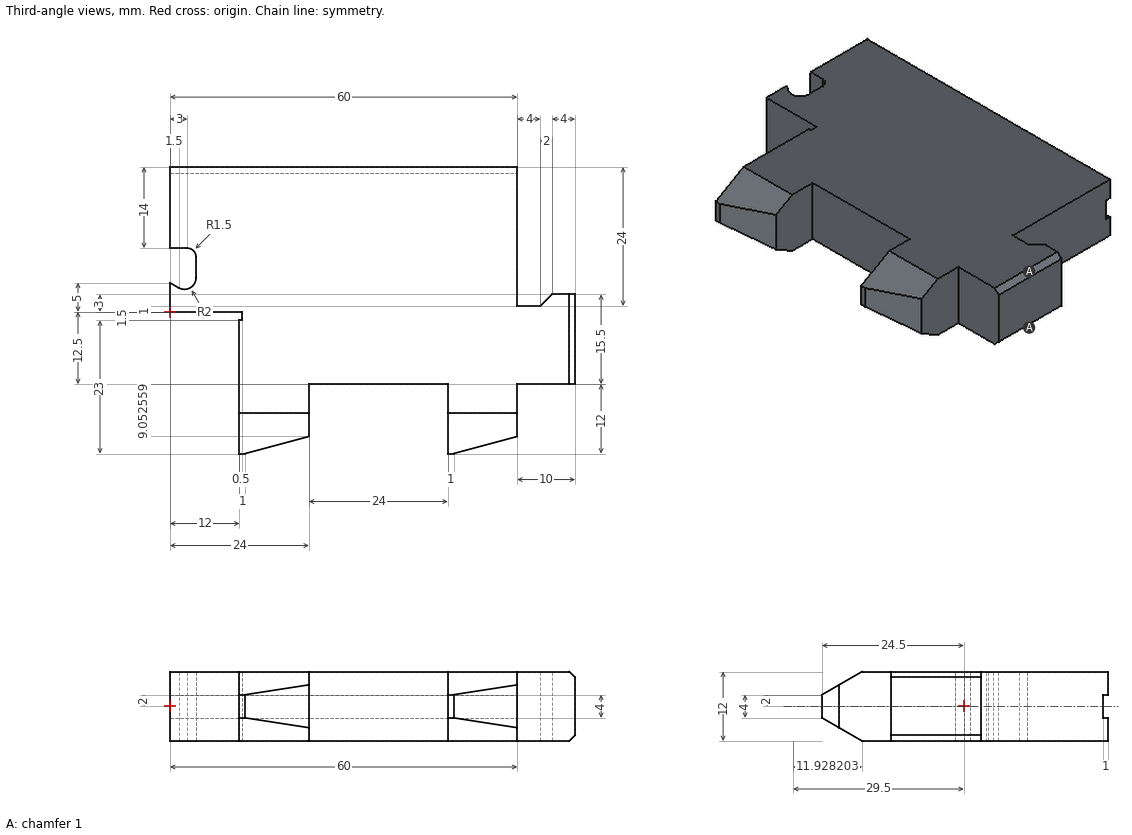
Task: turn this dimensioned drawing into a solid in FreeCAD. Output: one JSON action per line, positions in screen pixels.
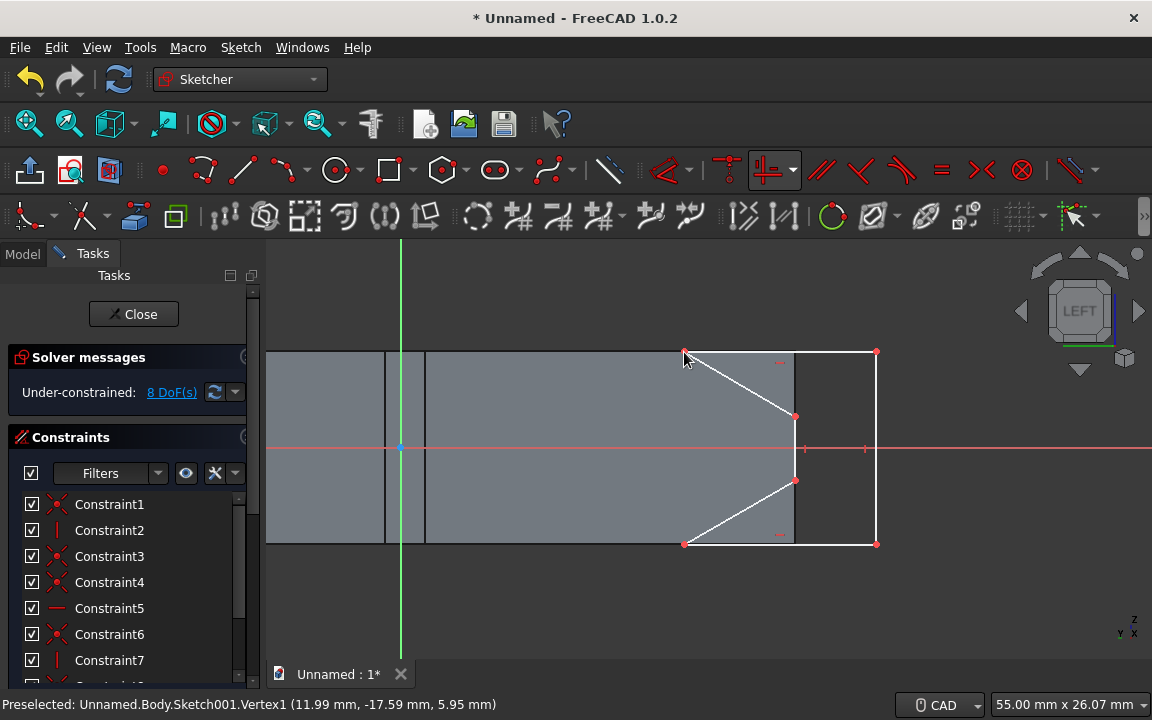
{"action": "left_click", "coordinate": [684, 352]}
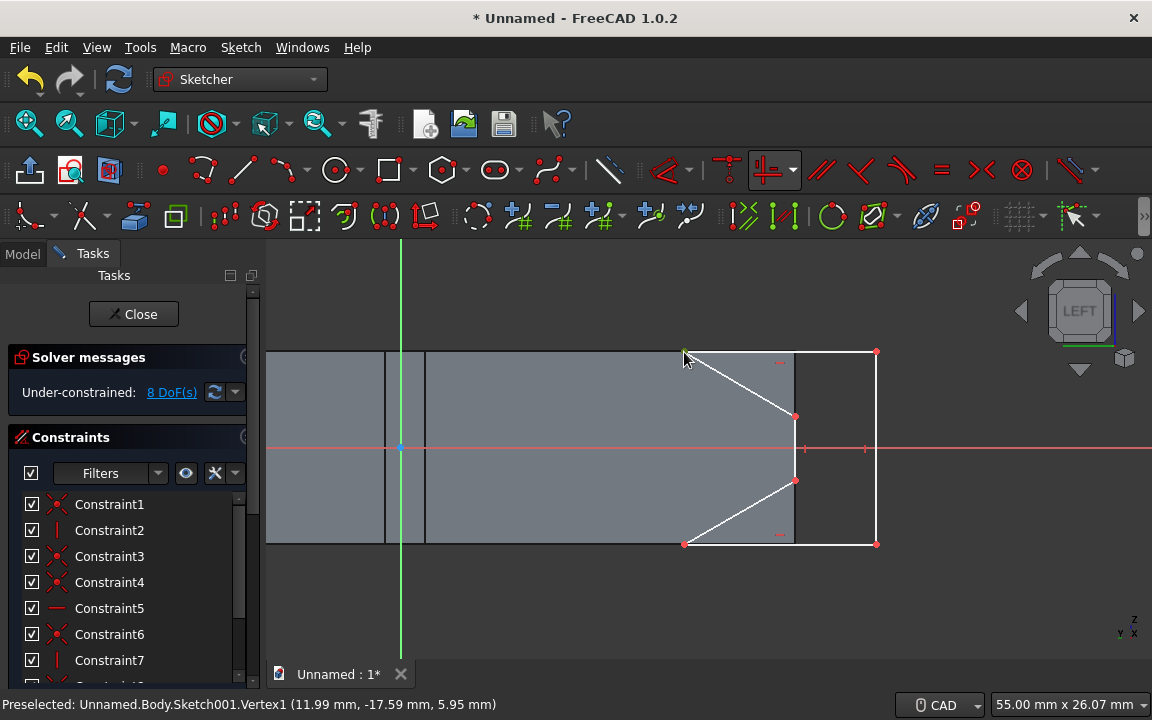
{"action": "left_click", "coordinate": [684, 545]}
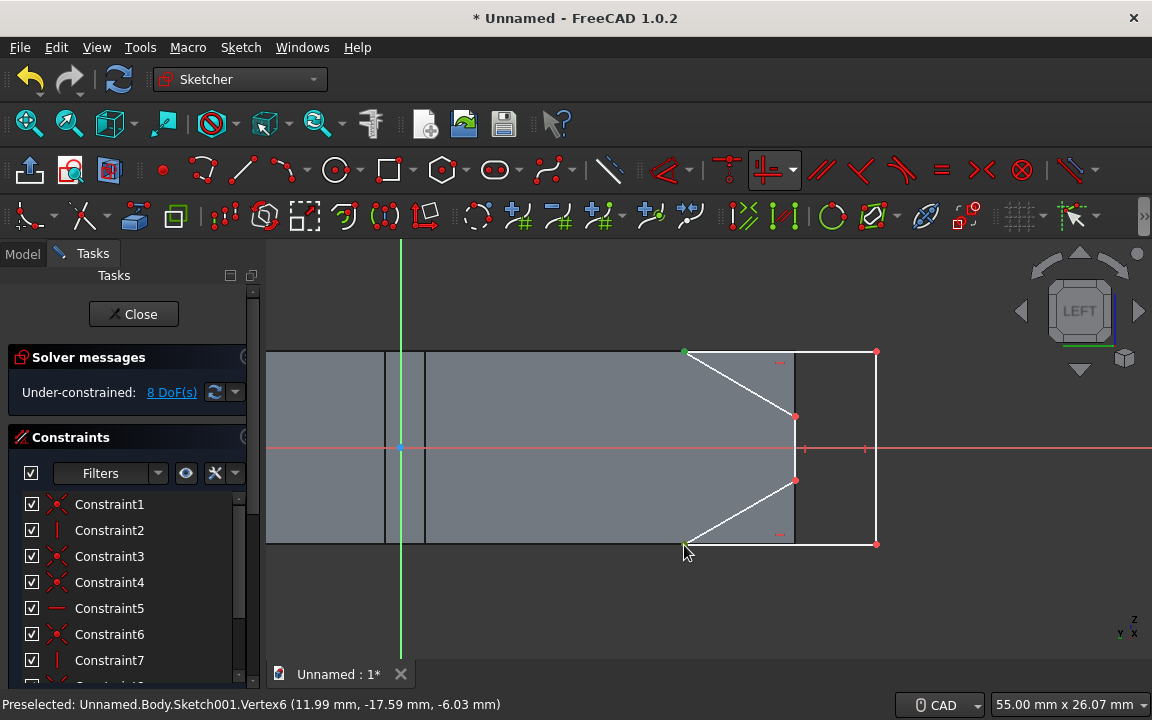
{"action": "left_click", "coordinate": [344, 448]}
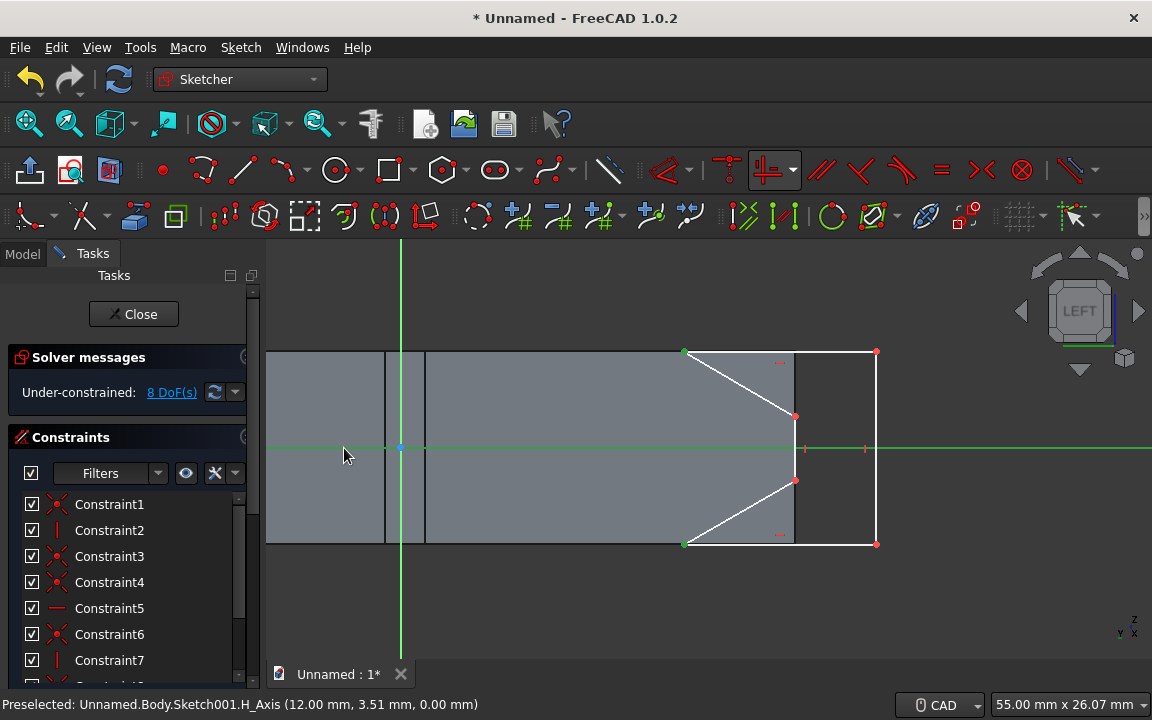
{"action": "left_click", "coordinate": [982, 170]}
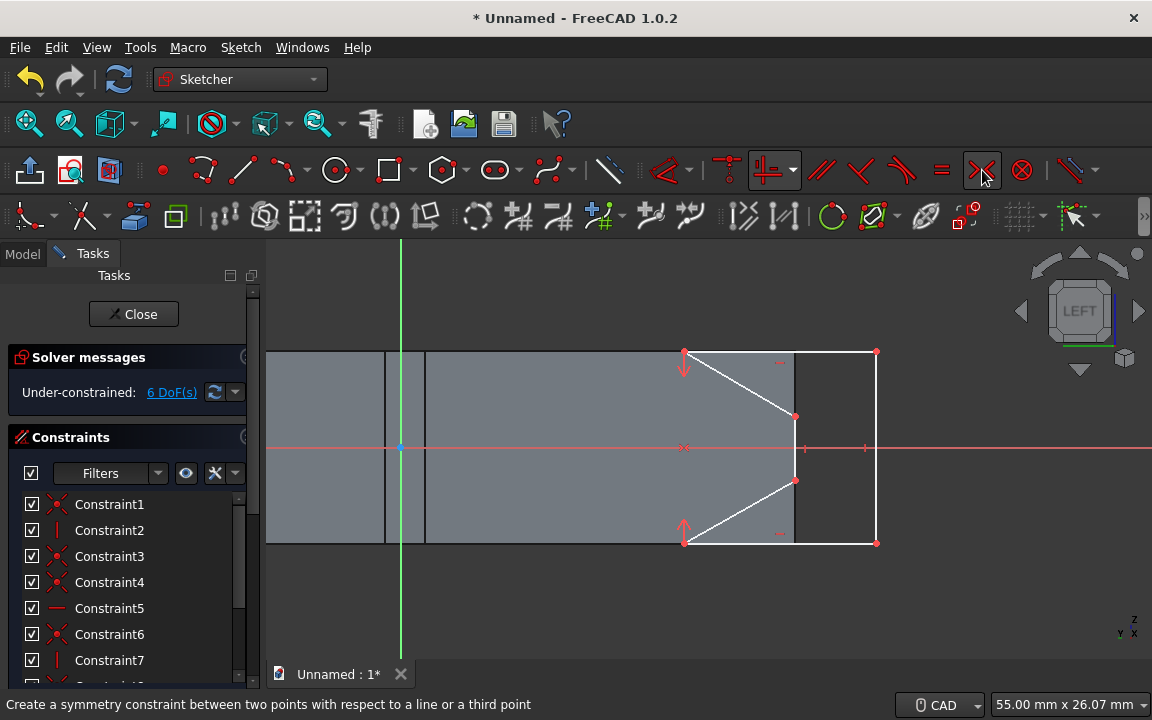
{"action": "left_click", "coordinate": [664, 170]}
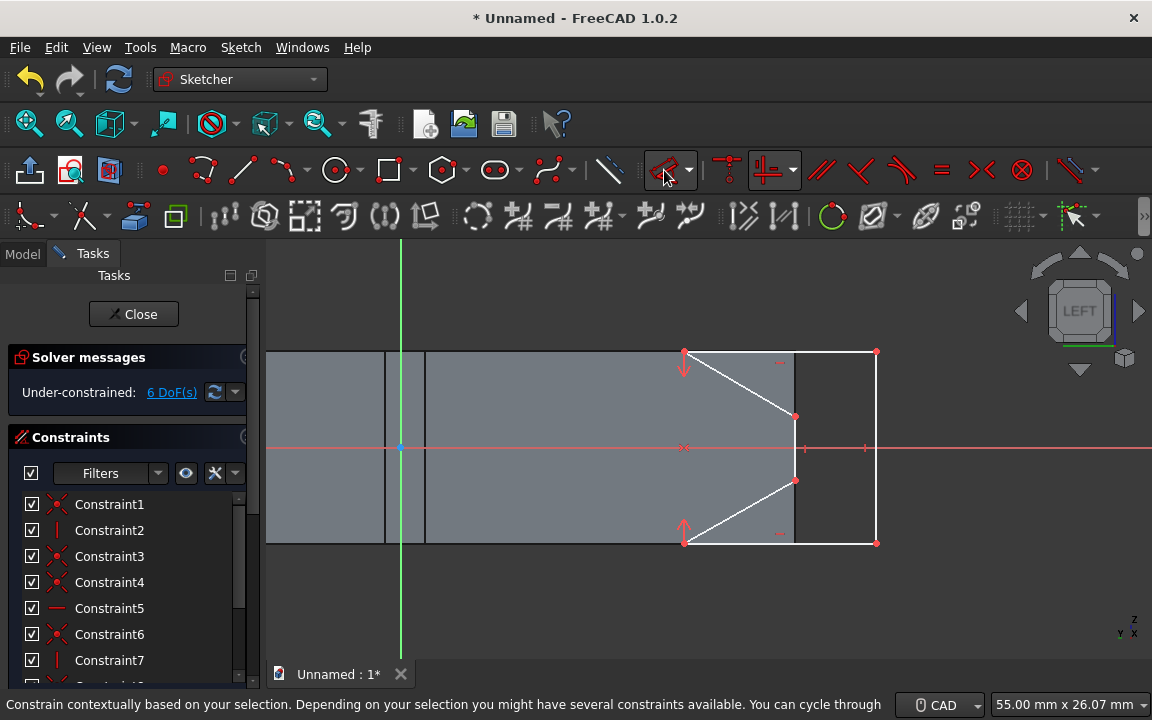
{"action": "left_click", "coordinate": [795, 436]}
{"action": "left_click", "coordinate": [829, 434]}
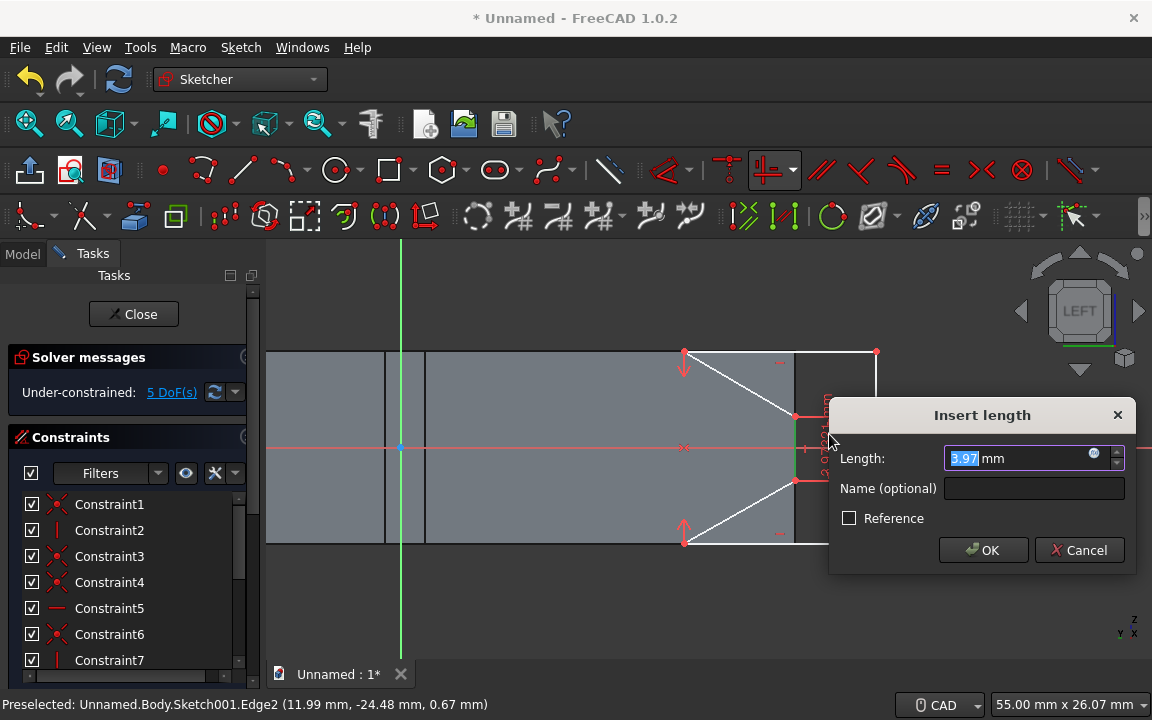
{"action": "type", "text": "4"}
{"action": "key", "text": "Return"}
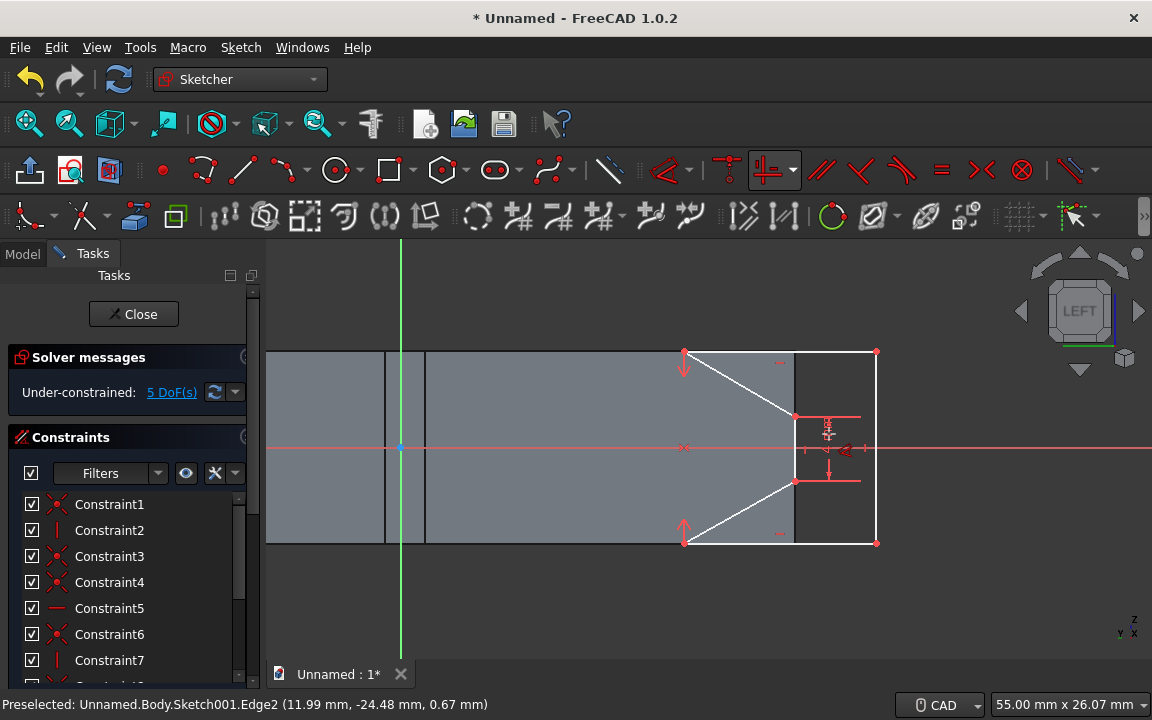
{"action": "left_click", "coordinate": [876, 486]}
{"action": "left_click", "coordinate": [910, 404]}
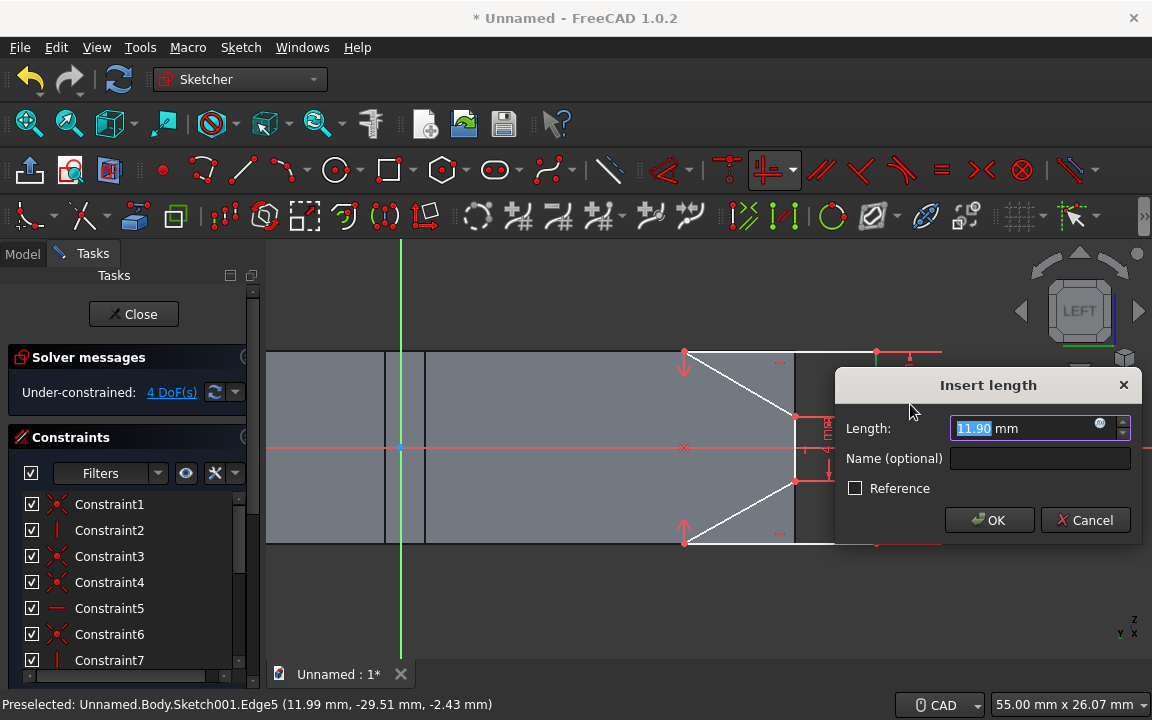
{"action": "type", "text": "12"}
{"action": "key", "text": "Return"}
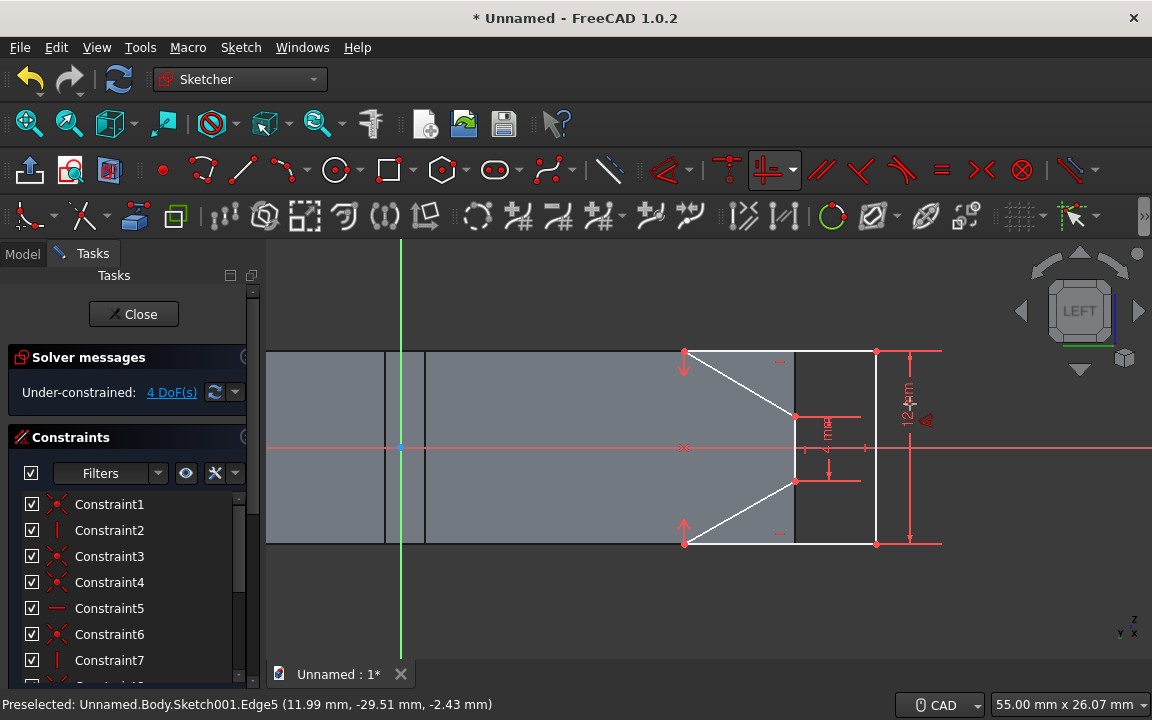
{"action": "scroll", "coordinate": [795, 417], "scroll_direction": "up", "scroll_amount": 2}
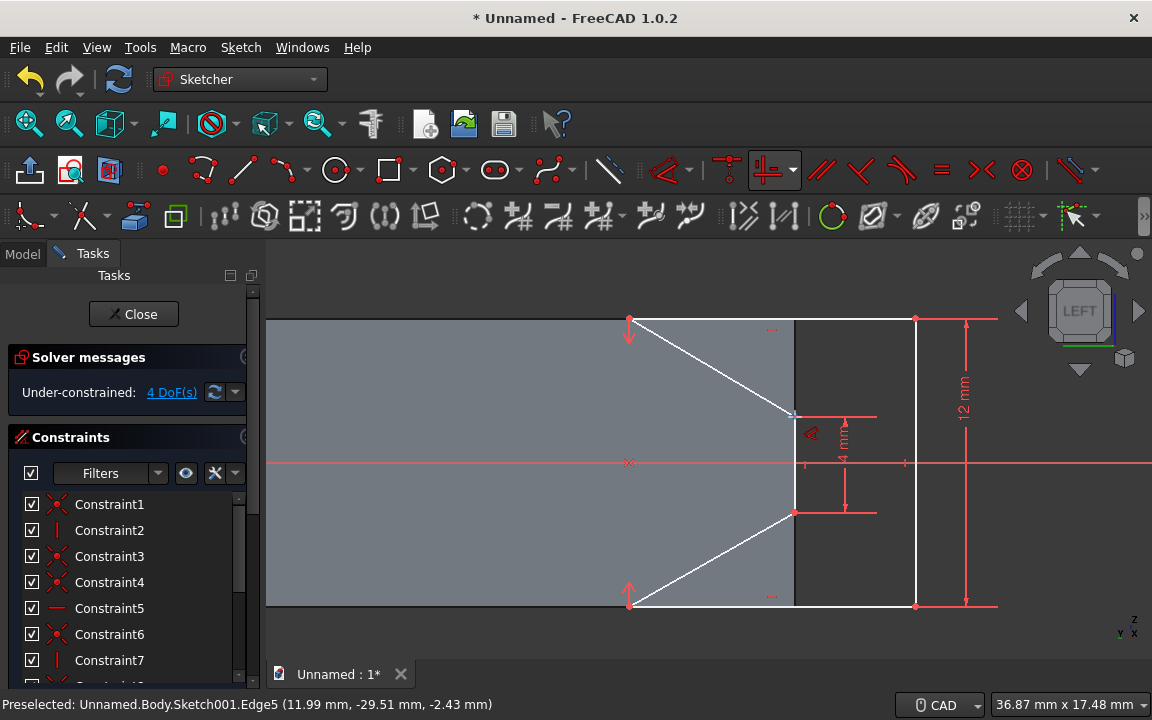
{"action": "left_click", "coordinate": [795, 417]}
{"action": "left_click", "coordinate": [949, 440]}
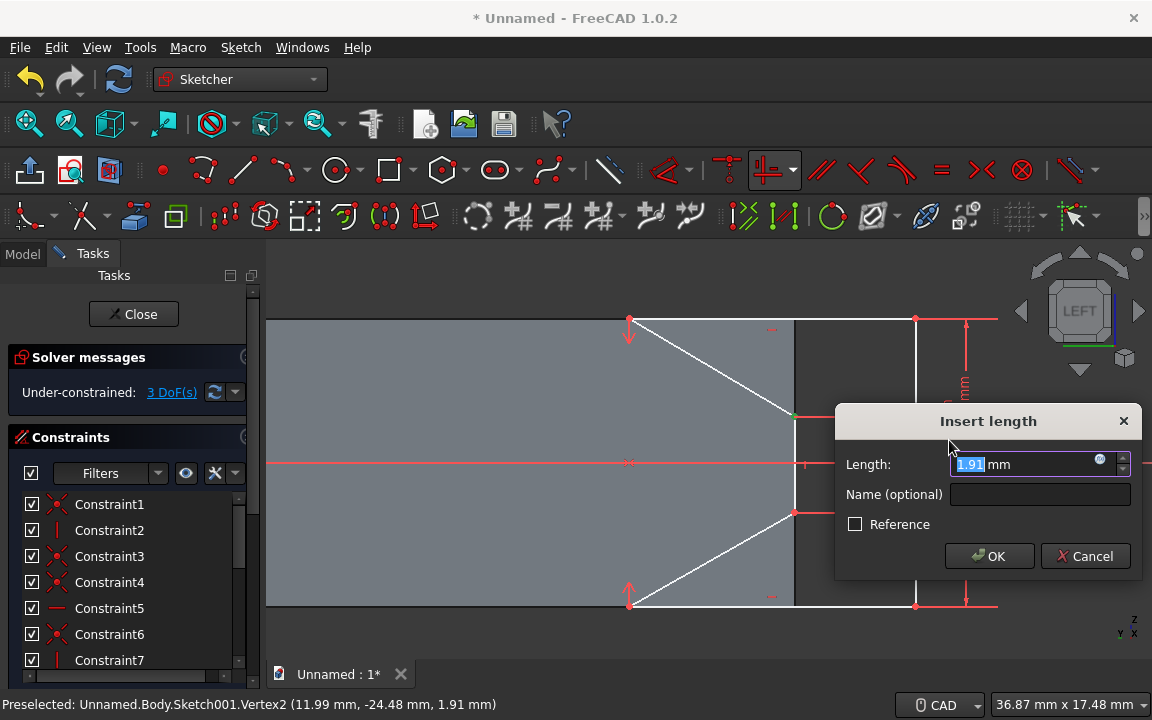
{"action": "type", "text": "2"}
{"action": "key", "text": "Return"}